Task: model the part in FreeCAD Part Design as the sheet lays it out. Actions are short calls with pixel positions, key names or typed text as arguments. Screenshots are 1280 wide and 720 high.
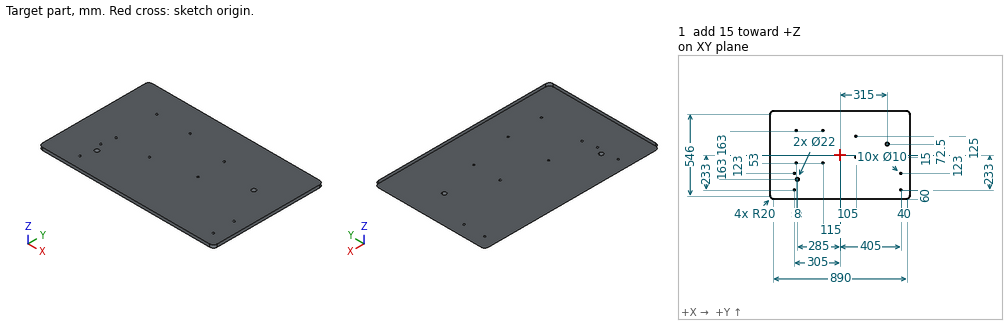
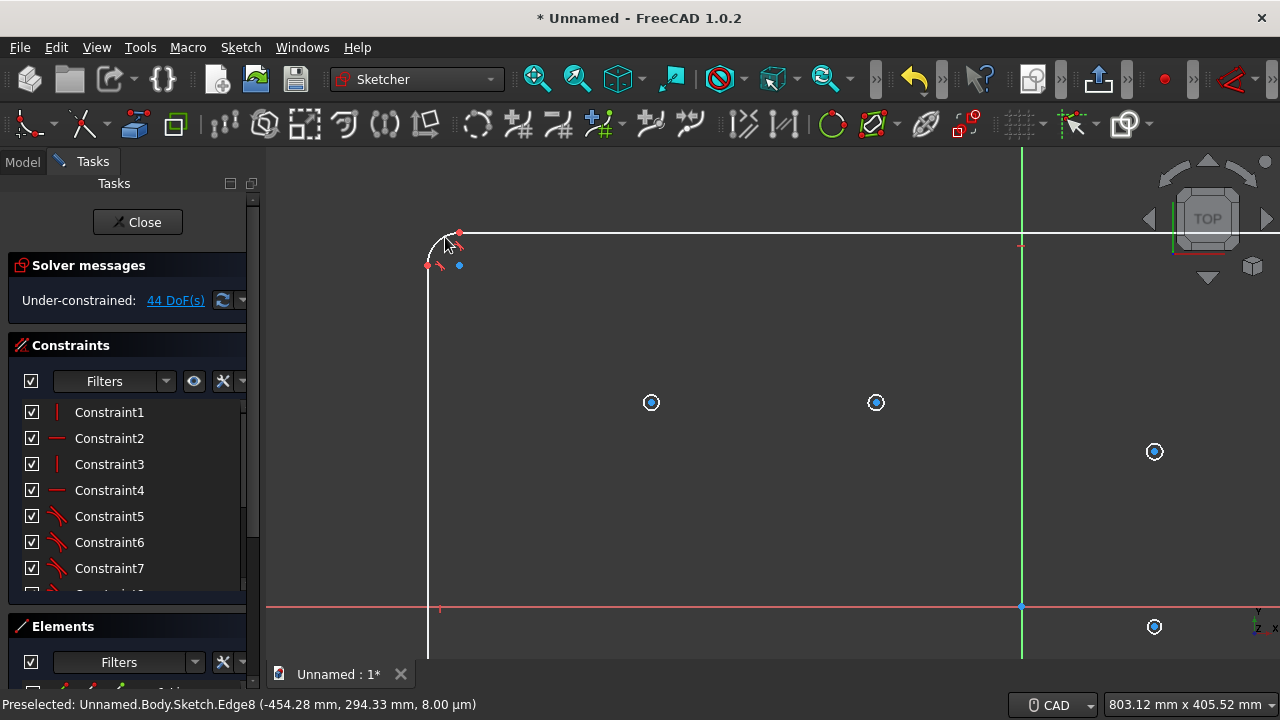
scroll(446, 237, down, 4)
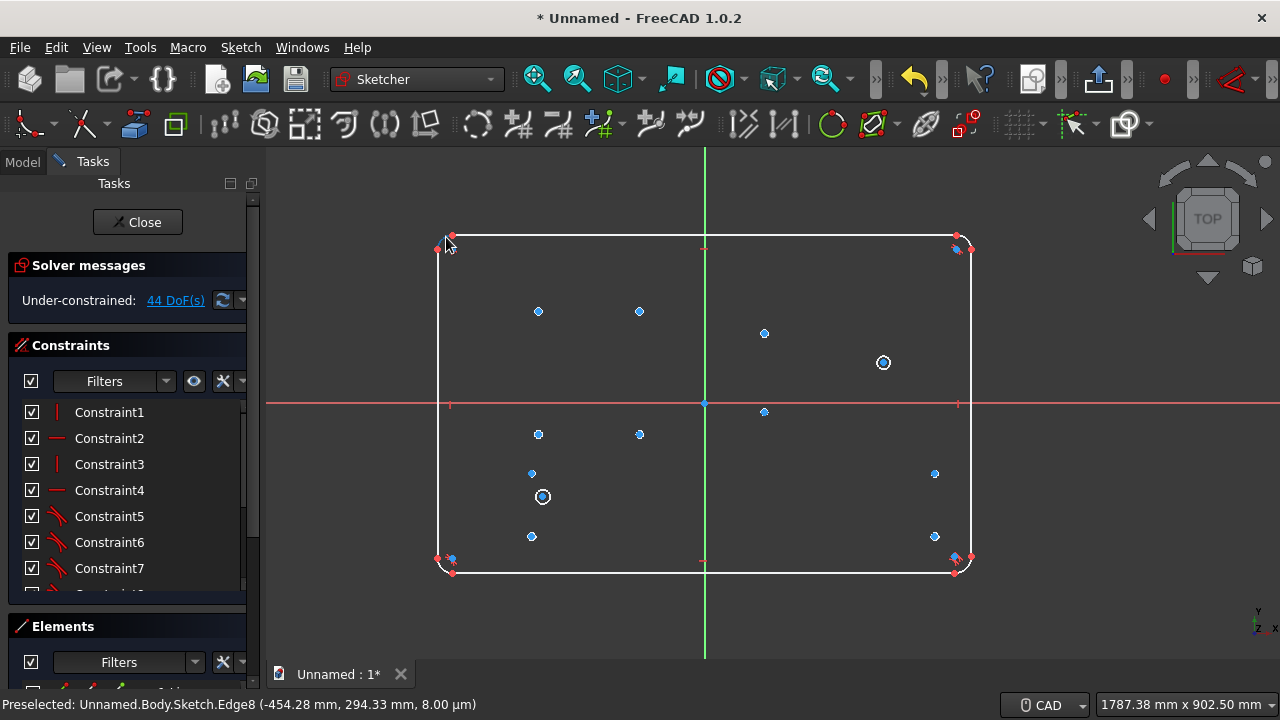
scroll(439, 565, up, 4)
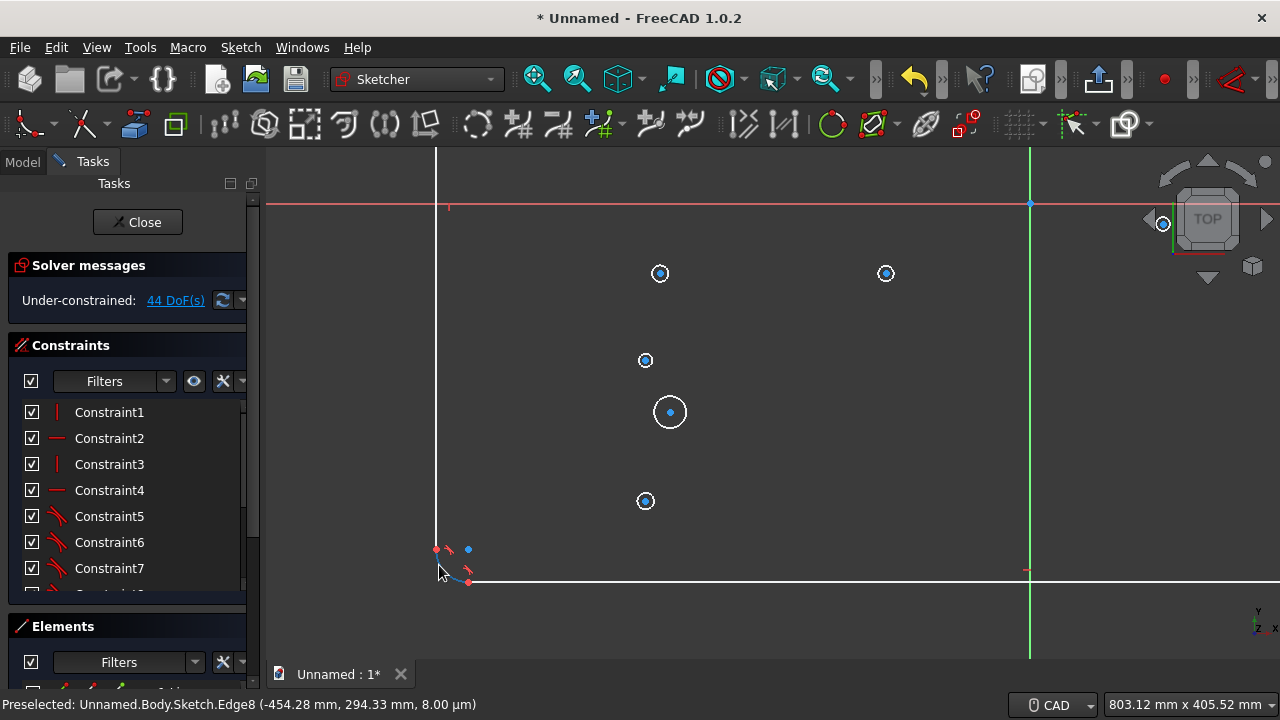
click(440, 565)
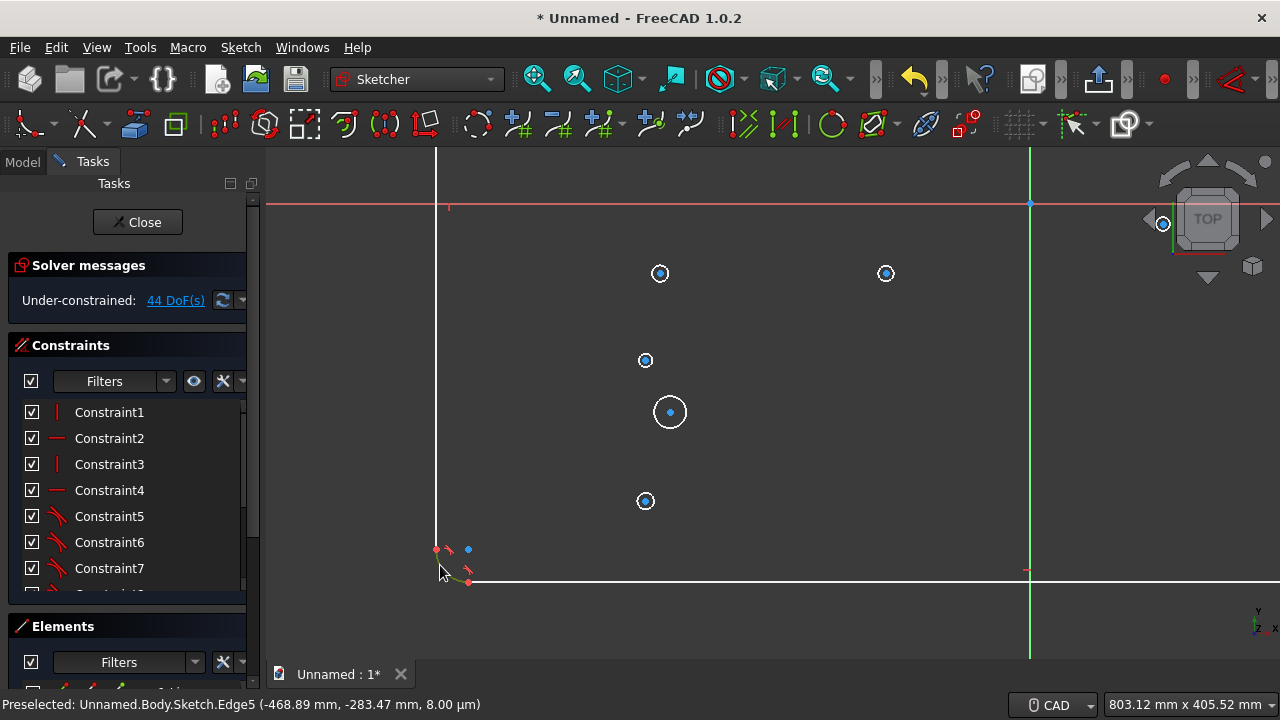
scroll(439, 565, down, 4)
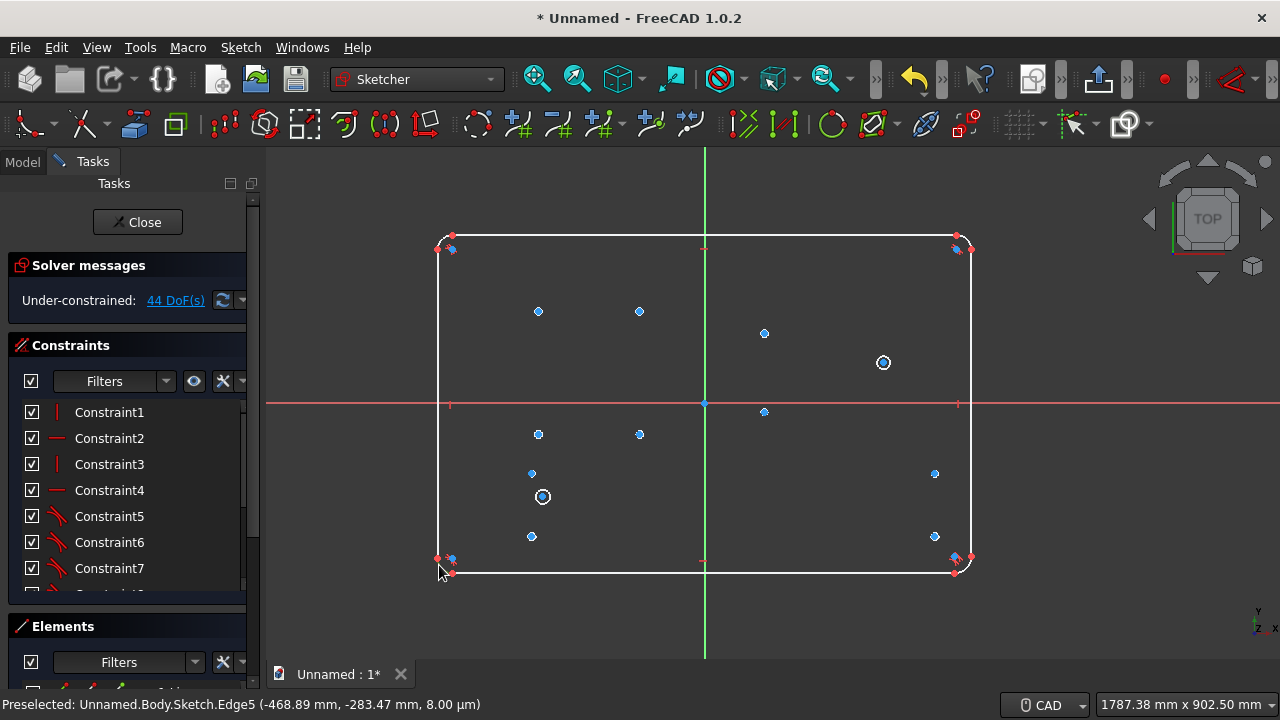
scroll(962, 571, up, 3)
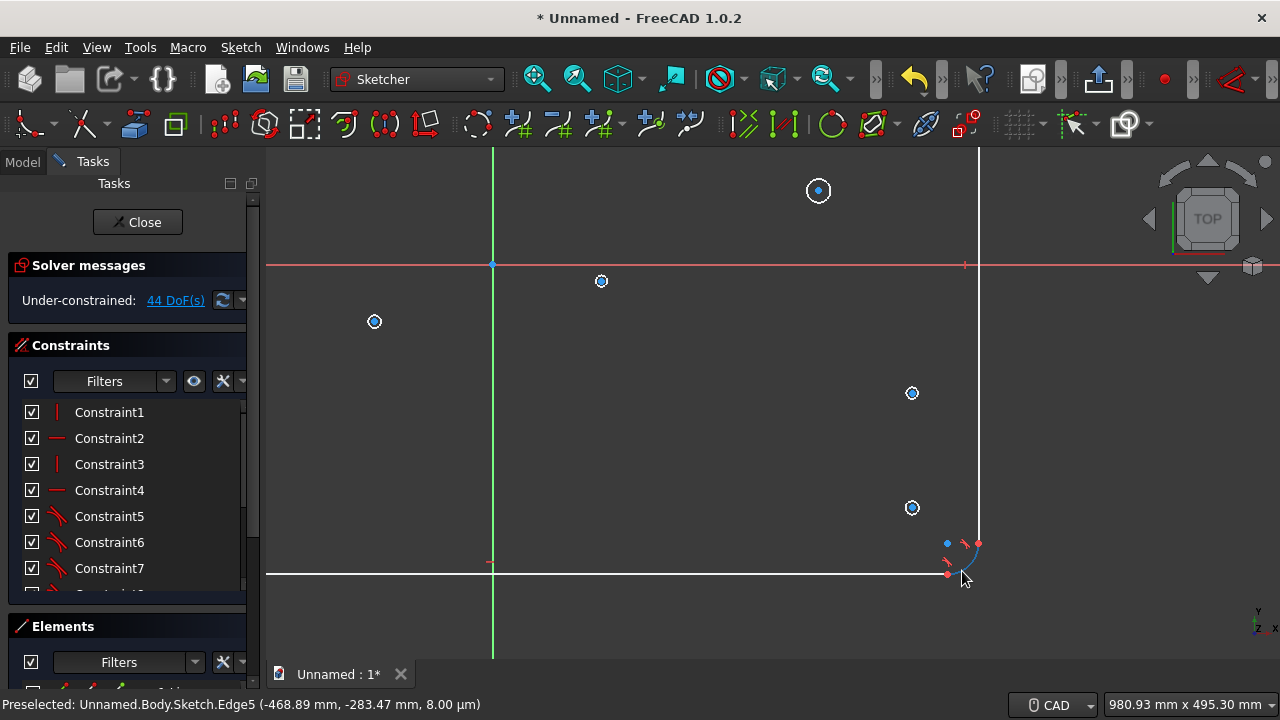
click(962, 571)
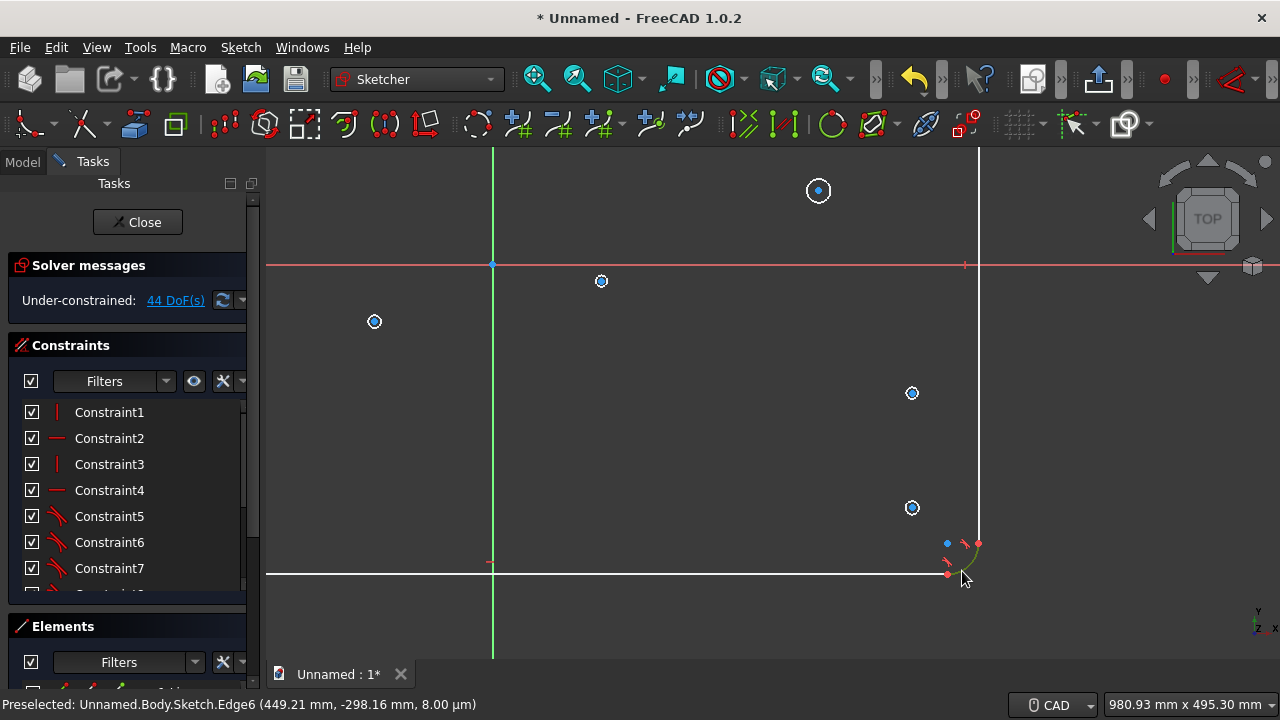
scroll(962, 571, down, 3)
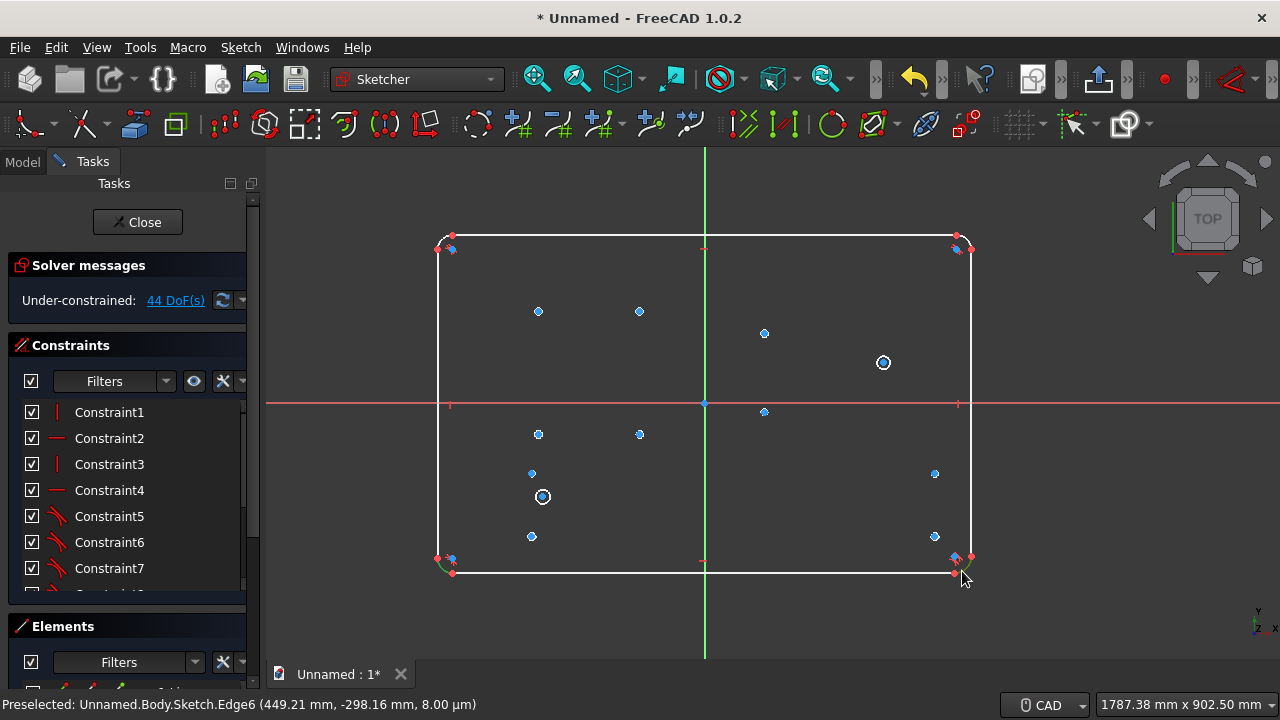
scroll(970, 243, up, 4)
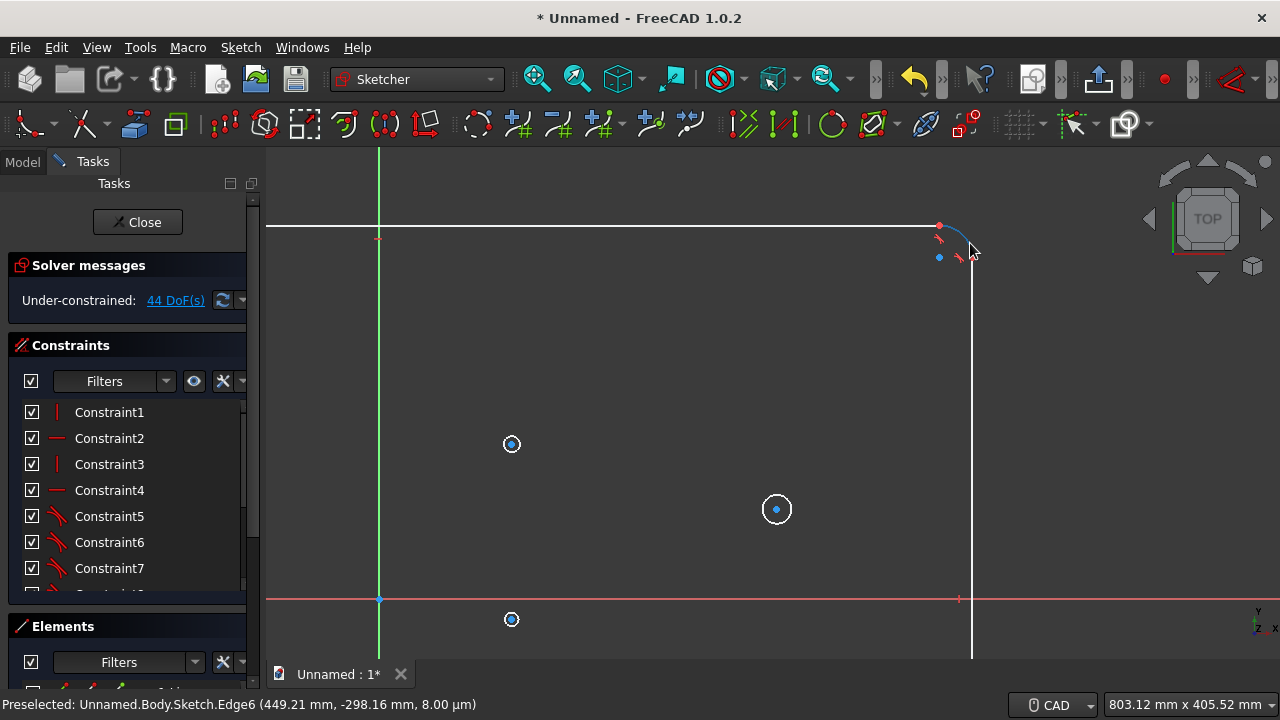
click(969, 243)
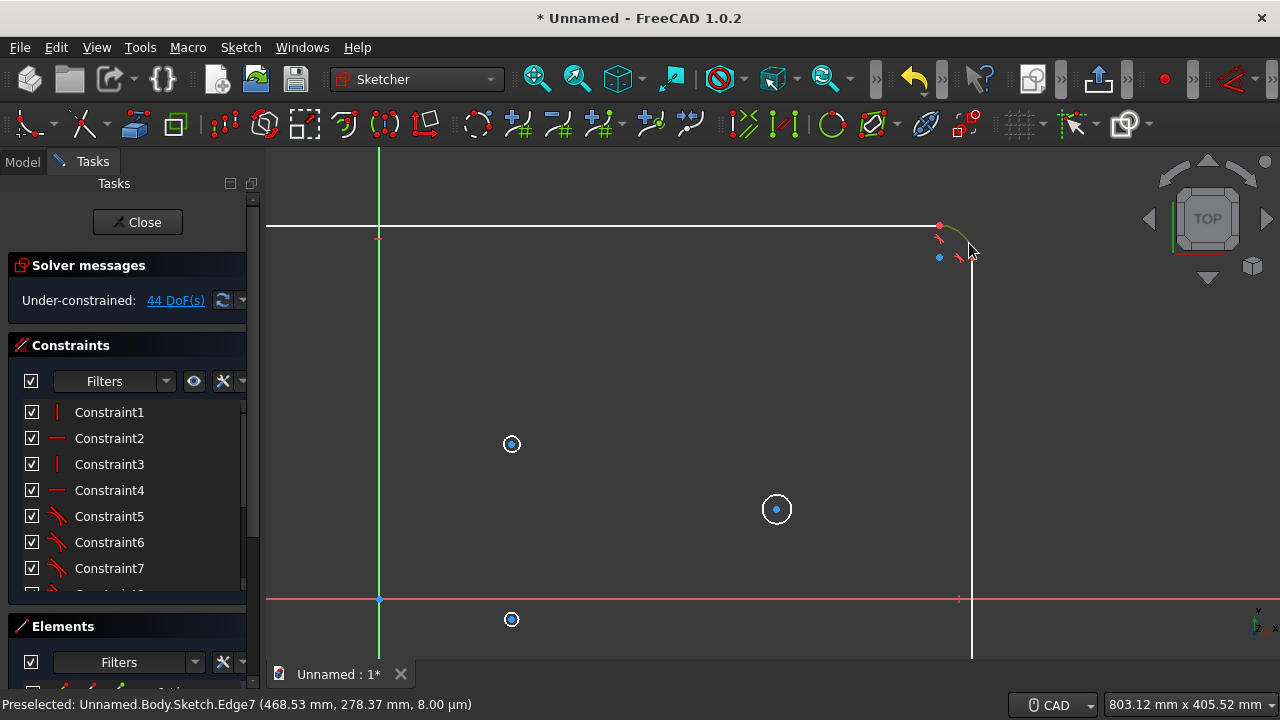
scroll(970, 243, down, 4)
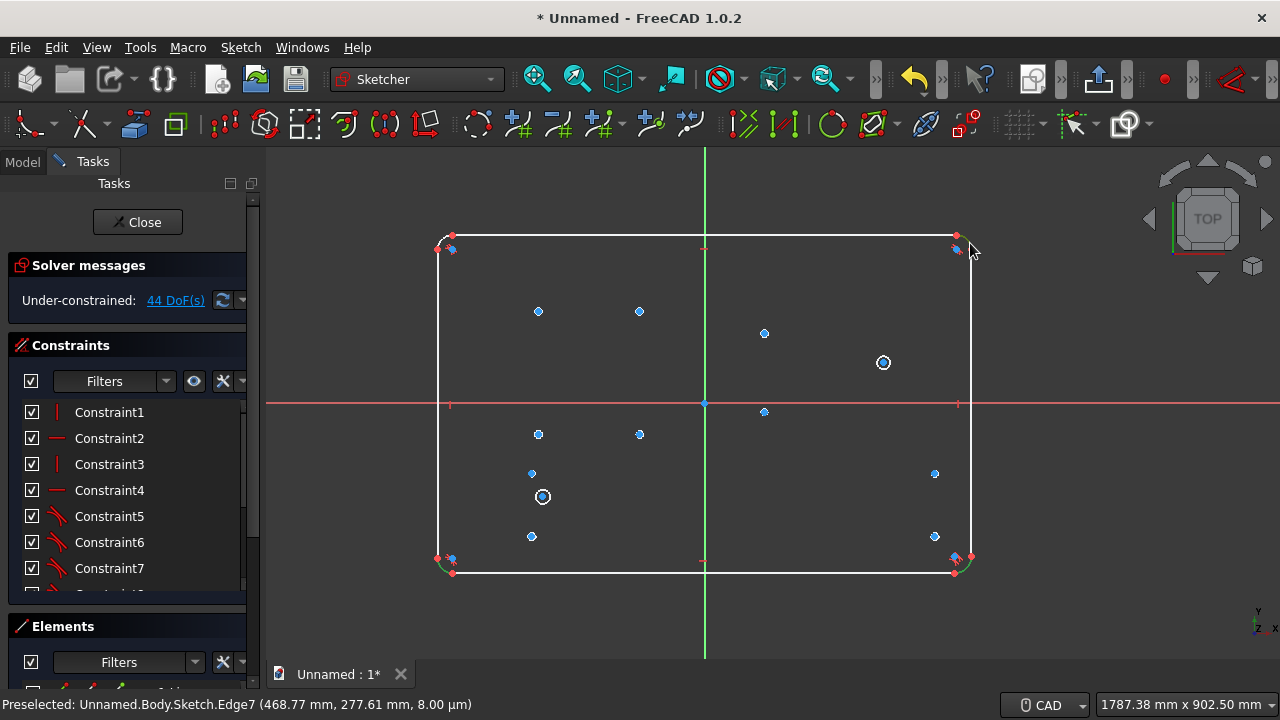
scroll(446, 237, up, 4)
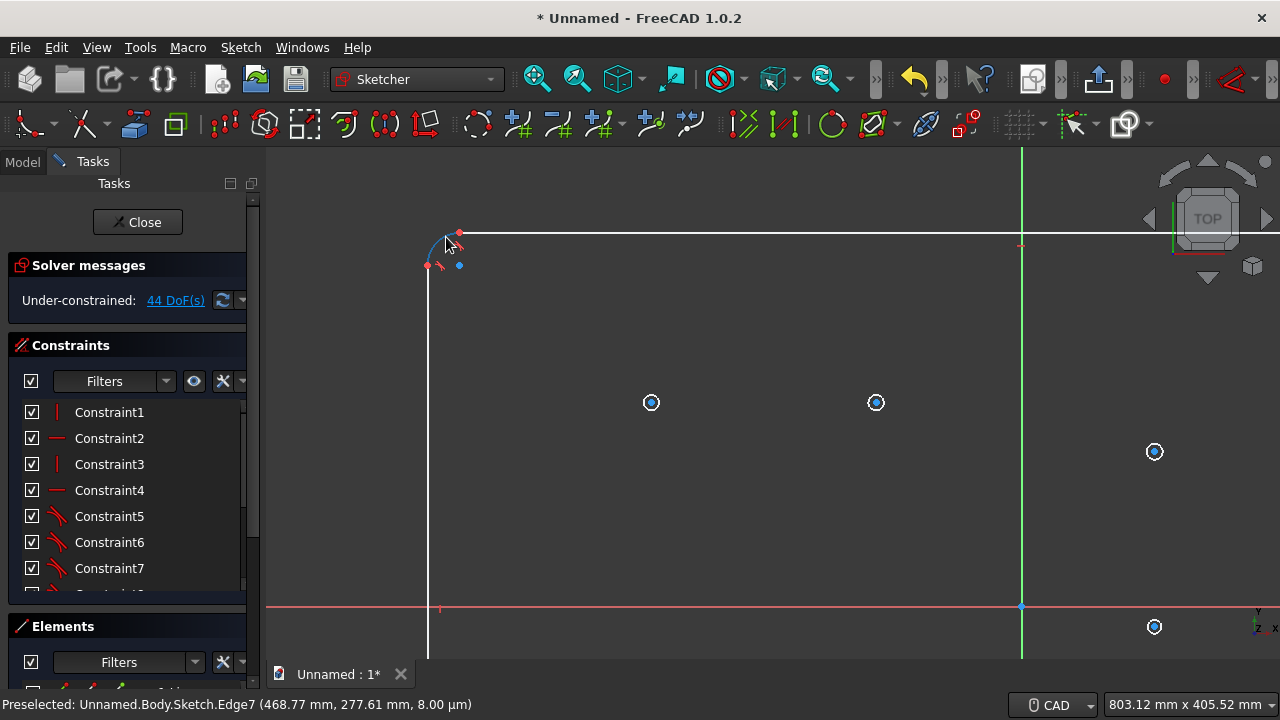
click(445, 236)